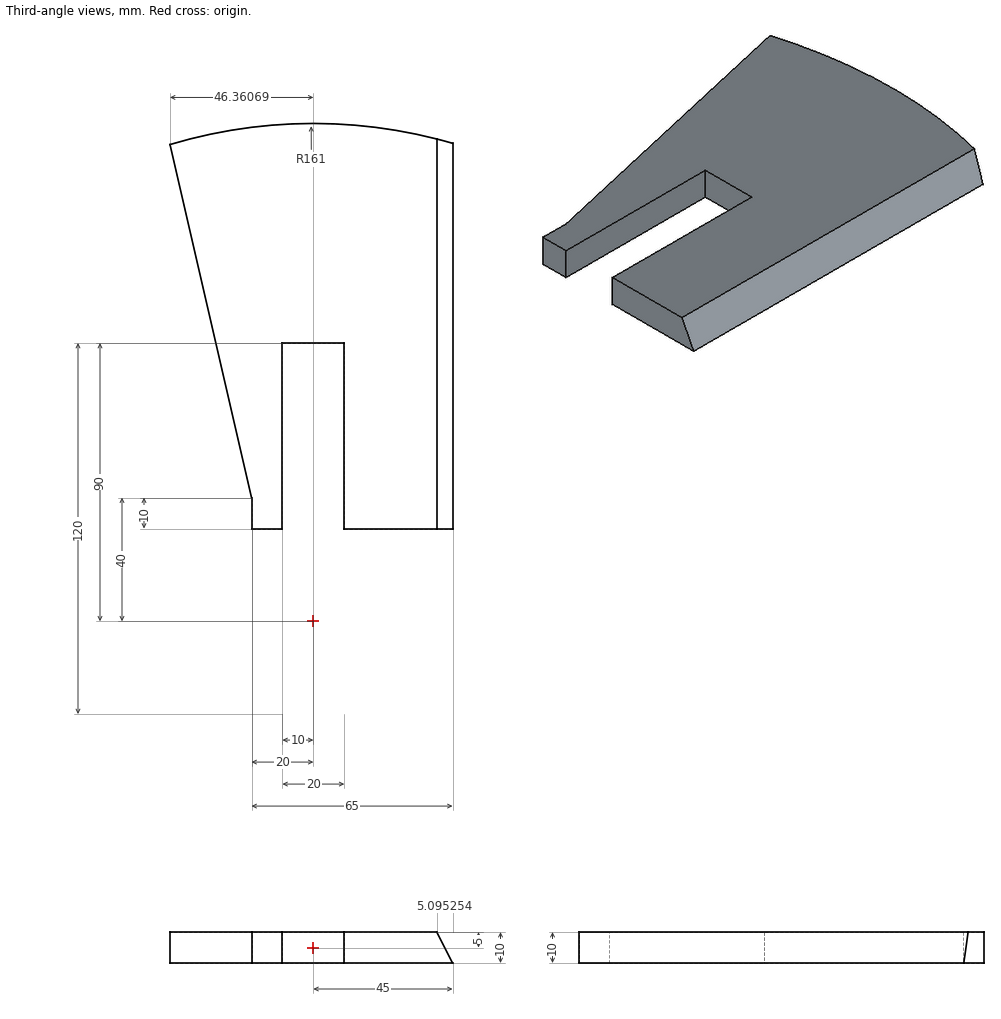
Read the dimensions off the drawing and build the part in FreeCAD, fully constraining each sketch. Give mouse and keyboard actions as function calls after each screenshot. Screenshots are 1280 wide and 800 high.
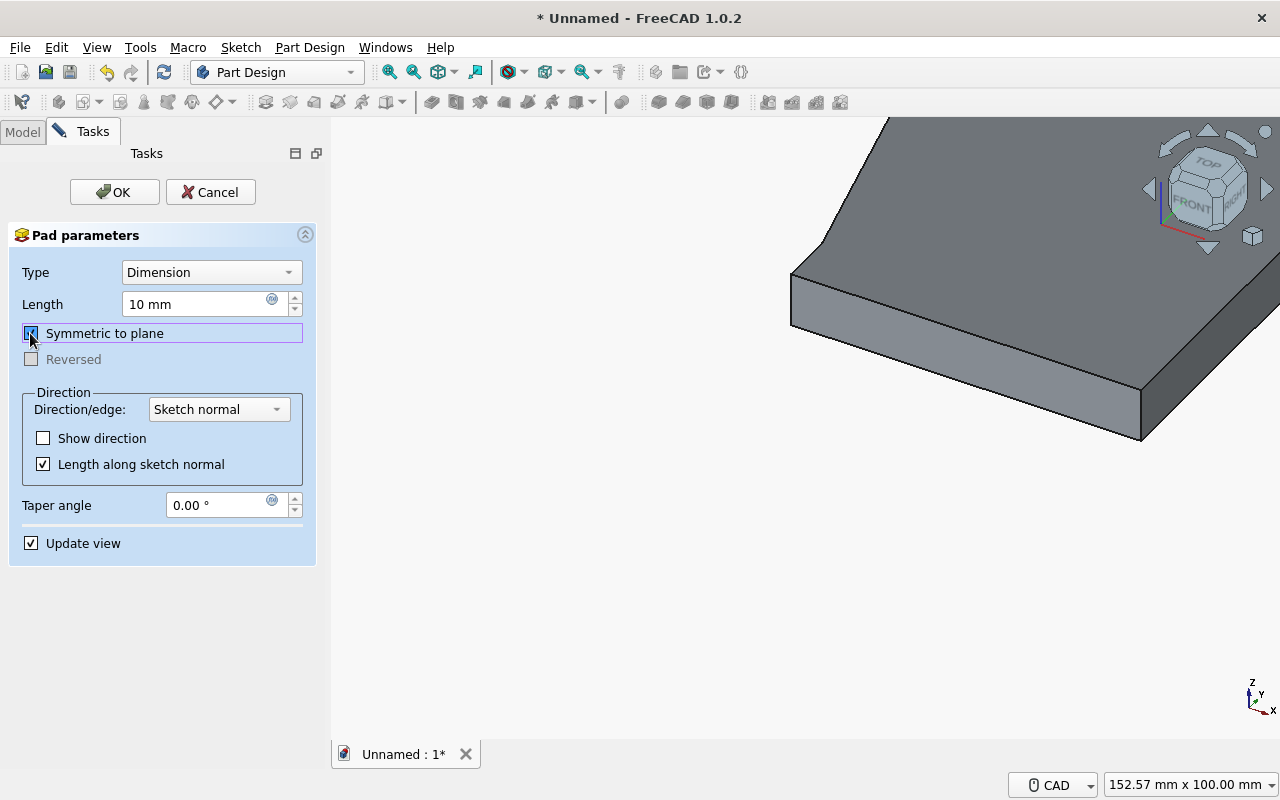
click(115, 192)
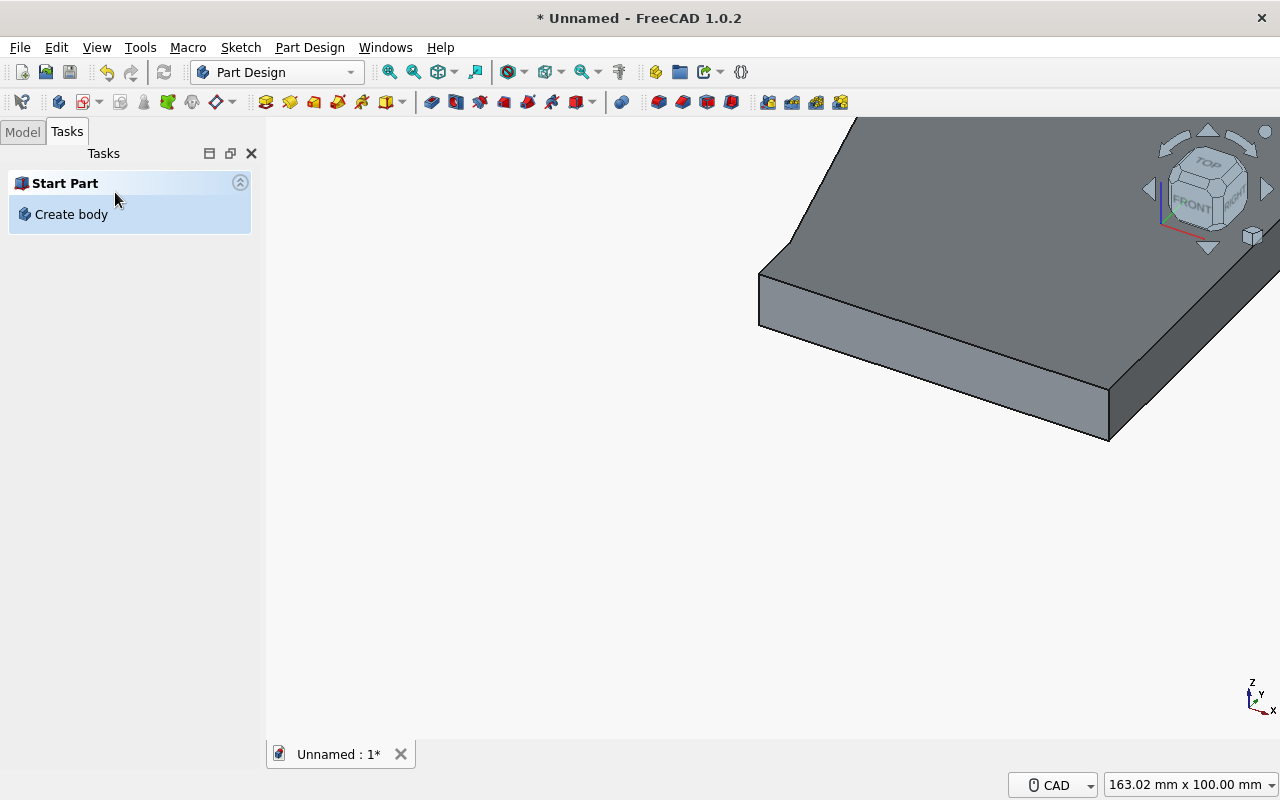
click(390, 72)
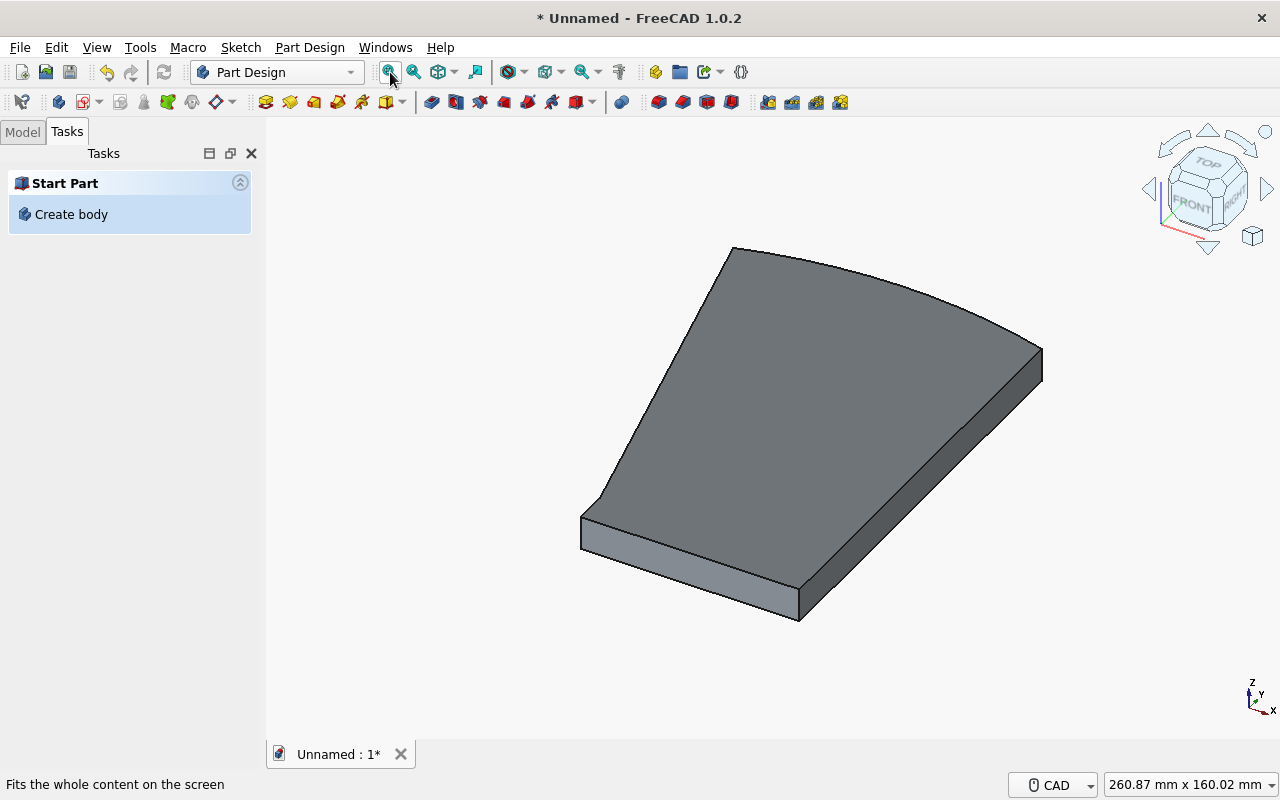
click(809, 375)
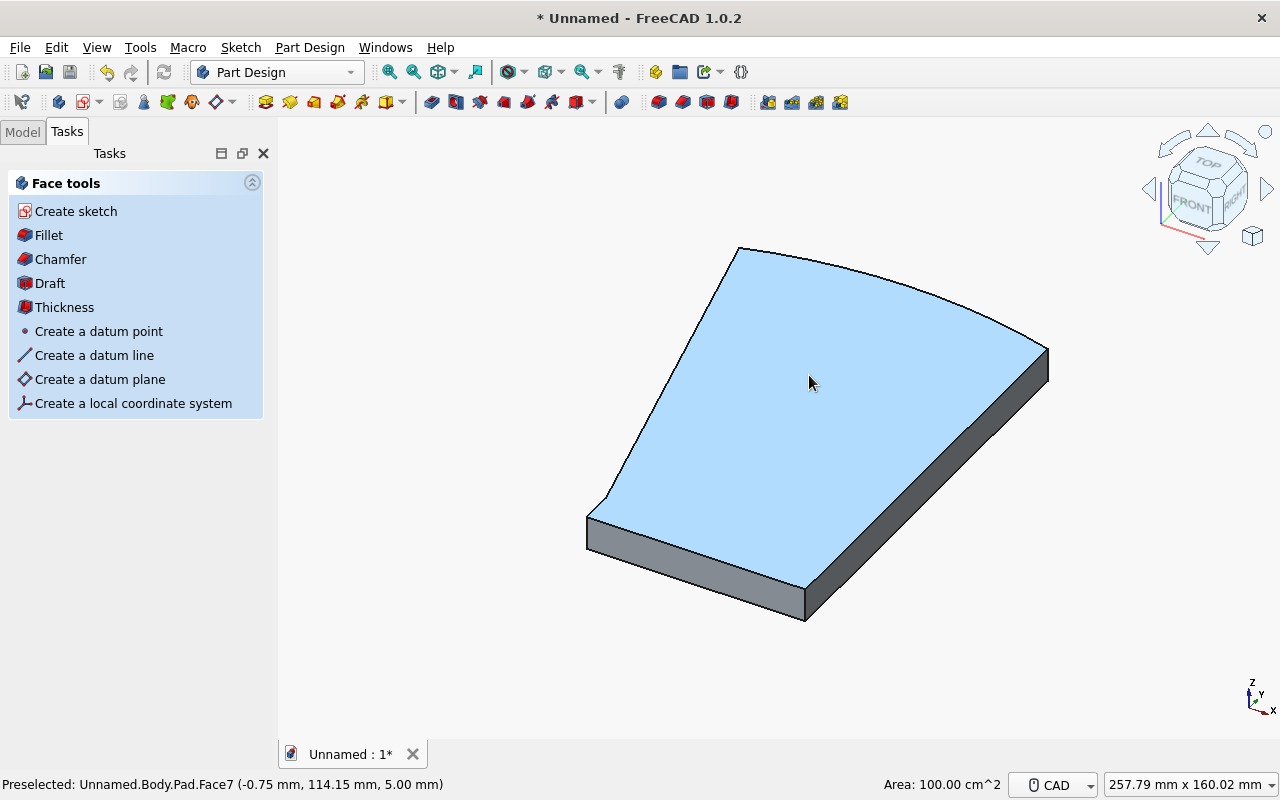
click(84, 102)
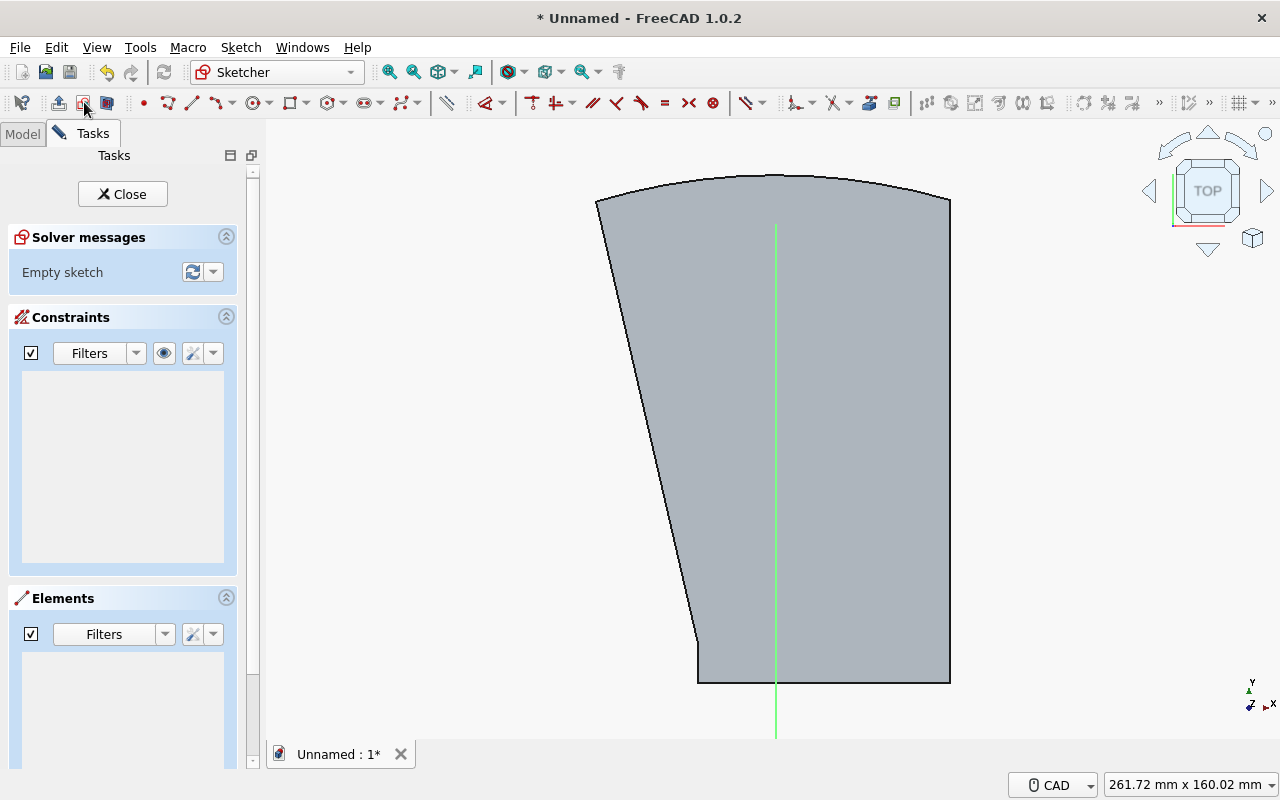
scroll(560, 147, down, 2)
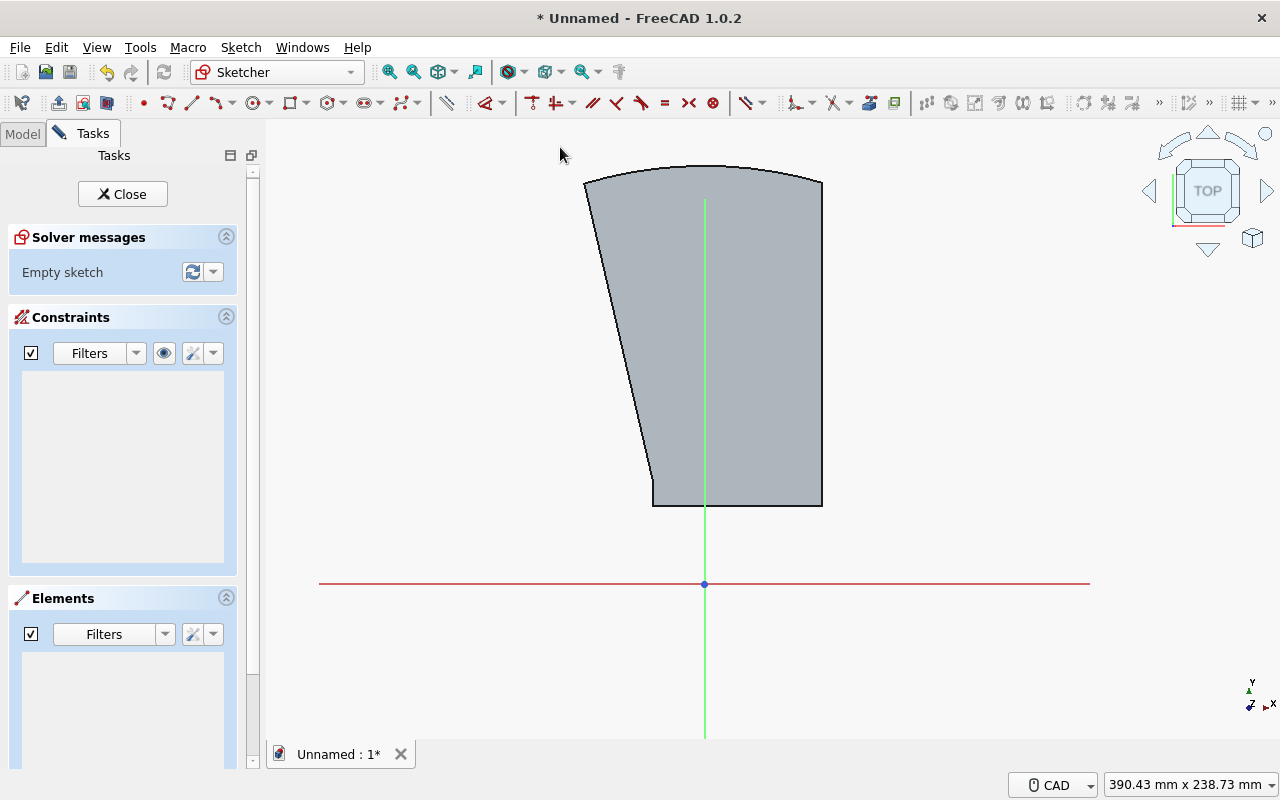
key(g)
key(r)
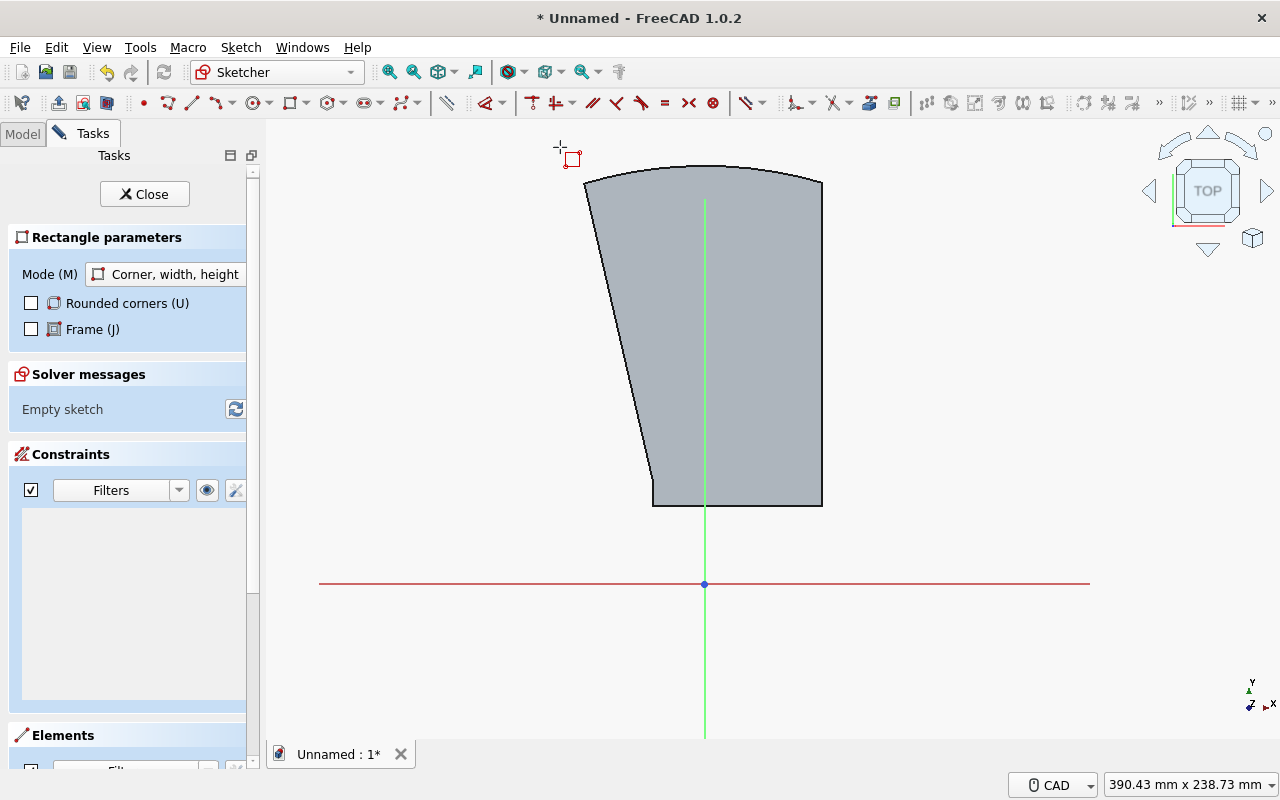
click(679, 350)
click(731, 662)
key(Escape)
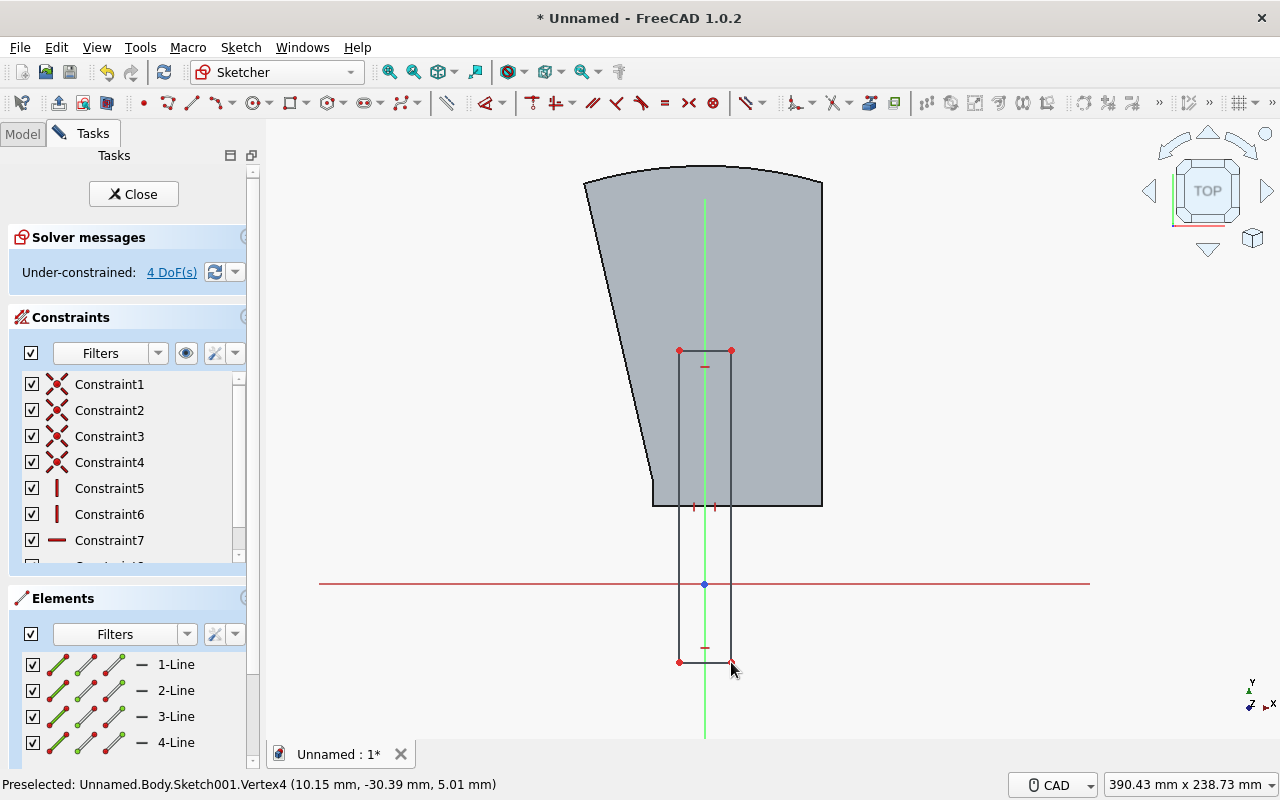
click(486, 104)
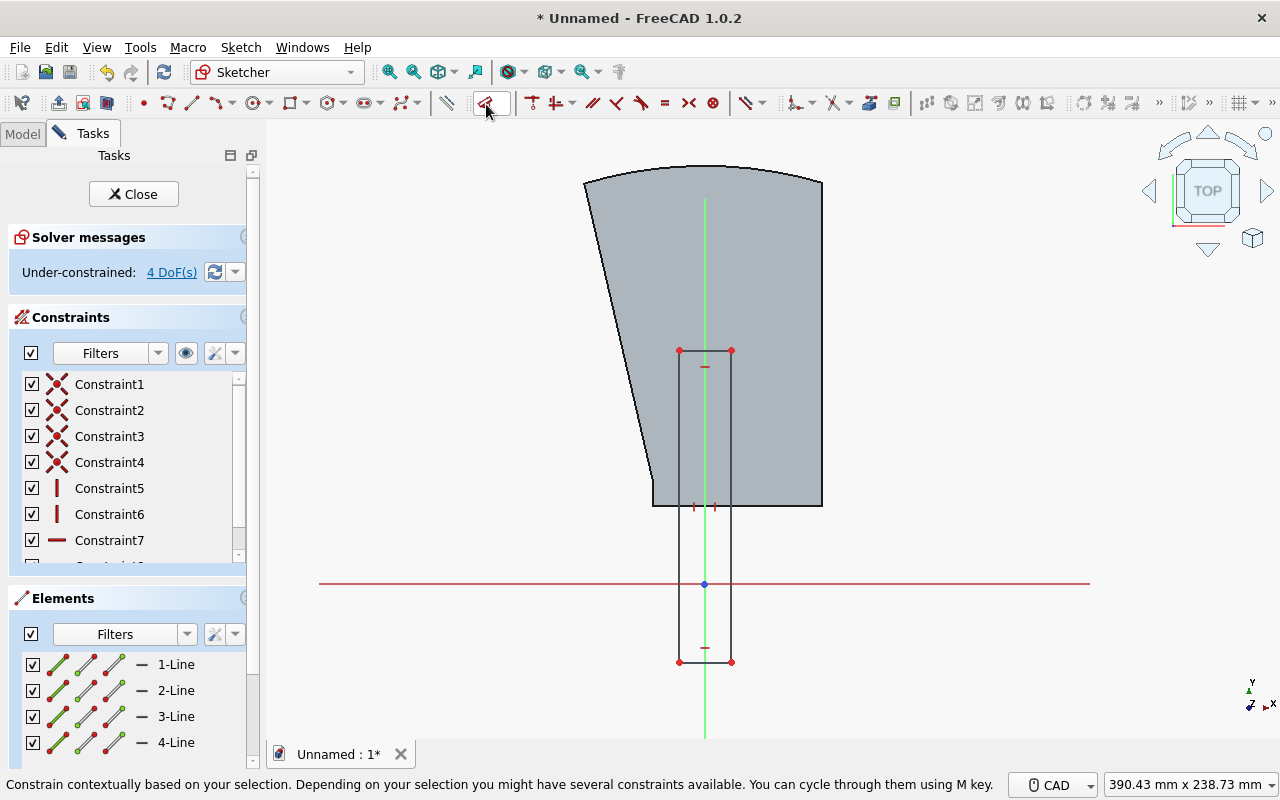
scroll(695, 663, up, 2)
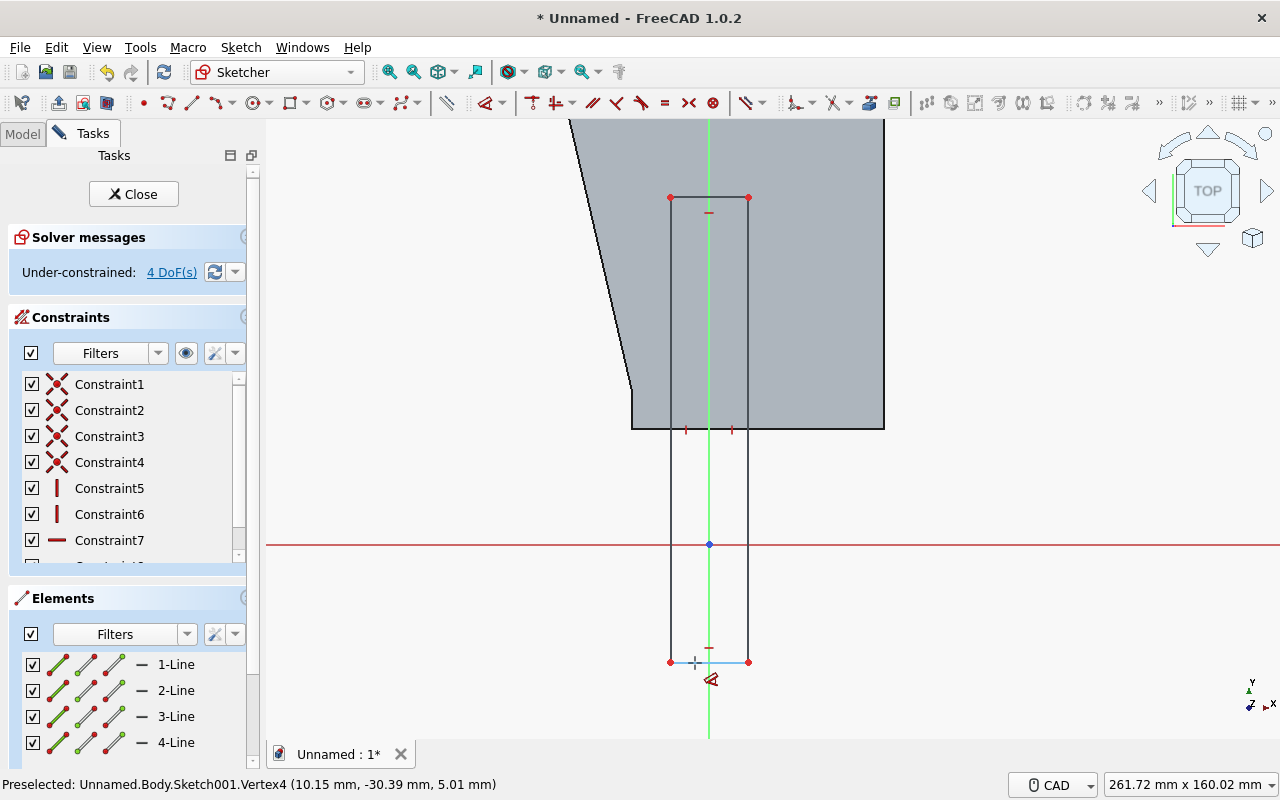
click(694, 663)
click(692, 697)